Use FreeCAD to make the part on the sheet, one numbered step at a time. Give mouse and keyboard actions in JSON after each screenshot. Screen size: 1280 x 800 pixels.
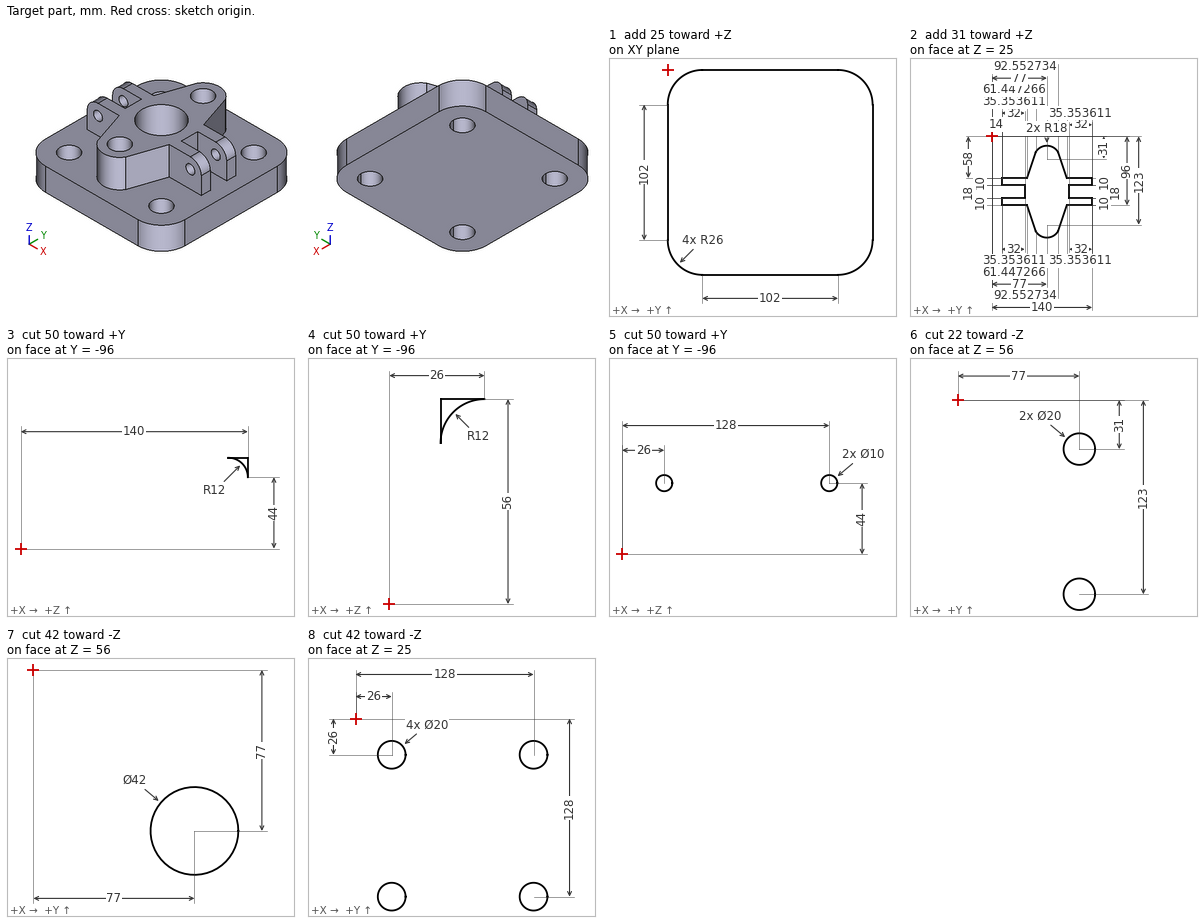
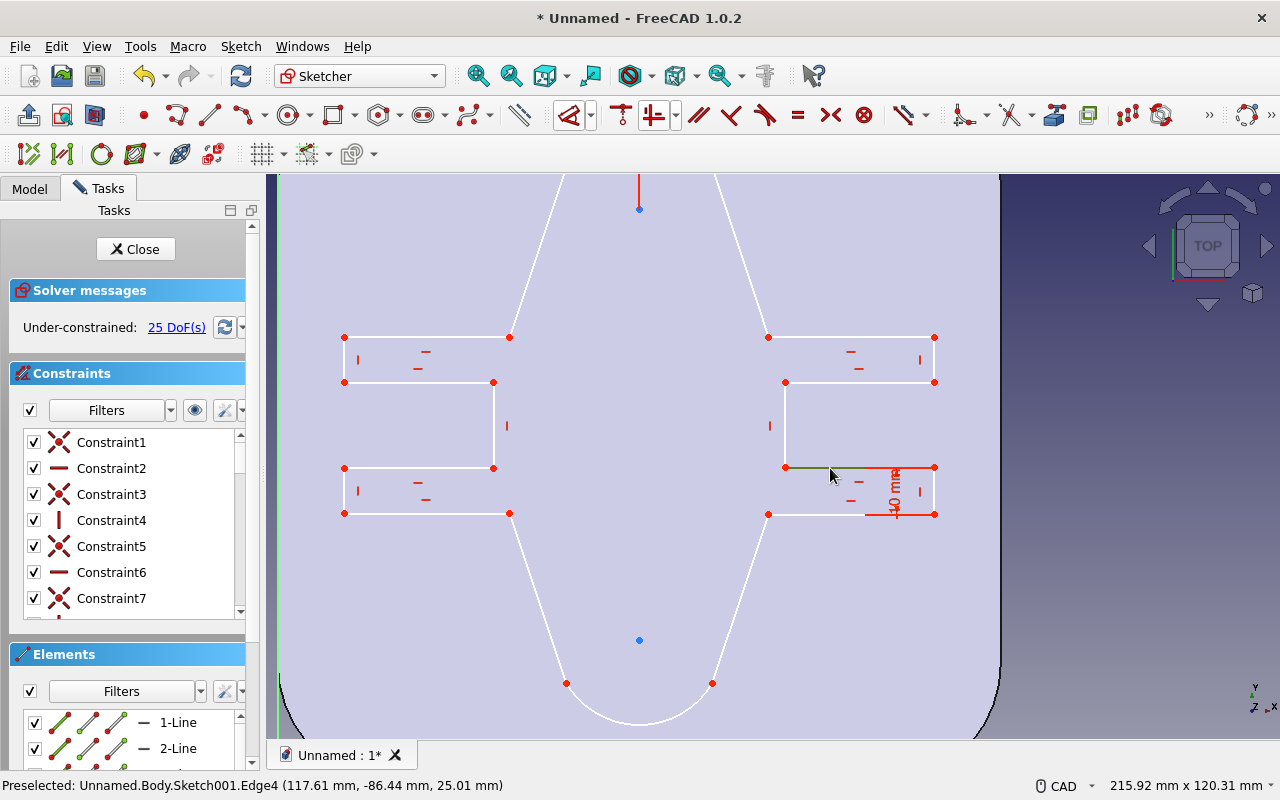
{"action": "key", "text": "l"}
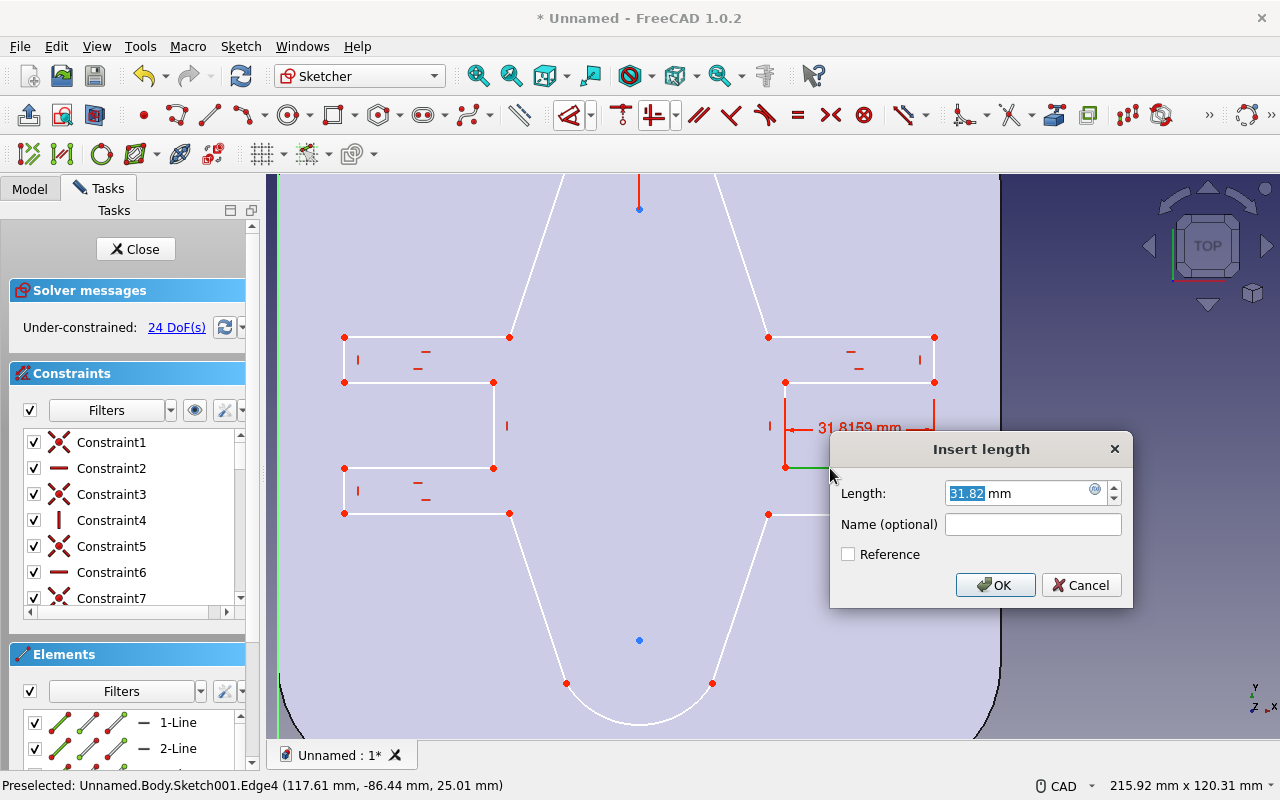
{"action": "type", "text": "32"}
{"action": "key", "text": "Return"}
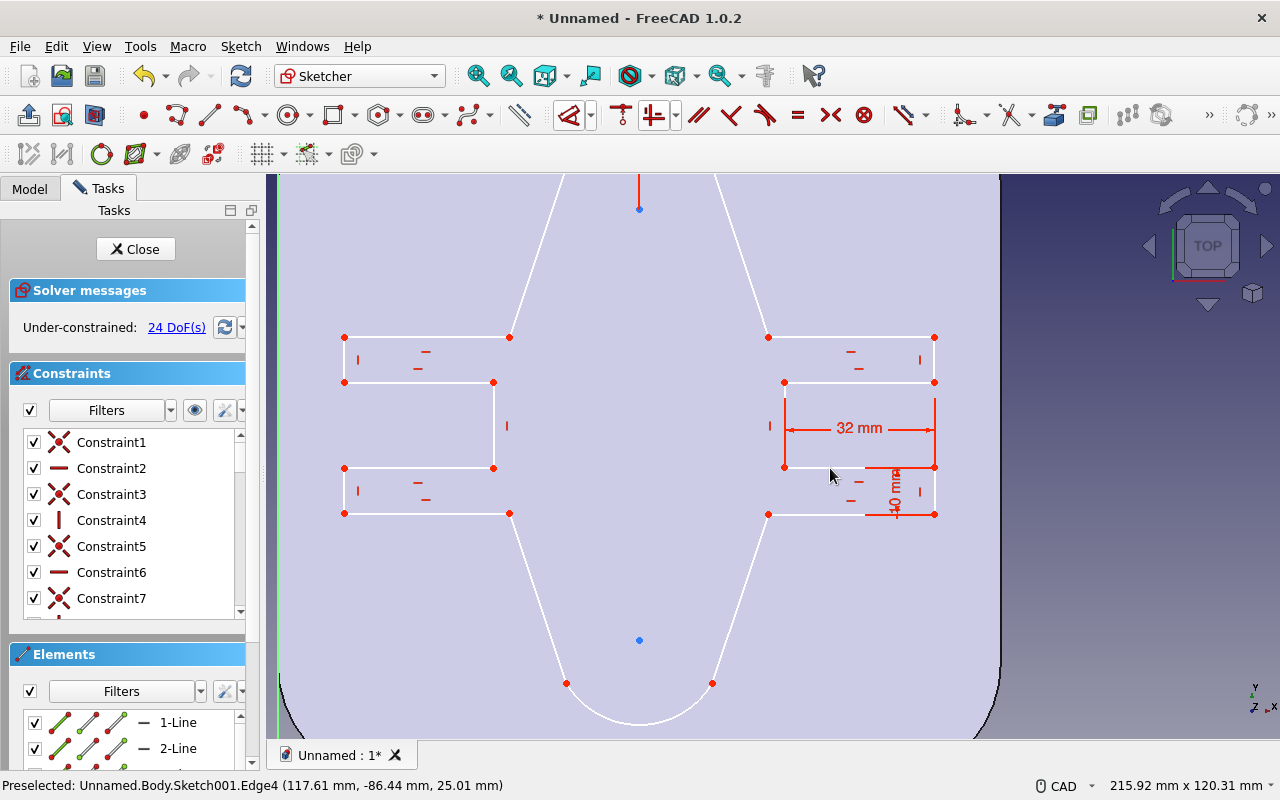
{"action": "left_click", "coordinate": [785, 442]}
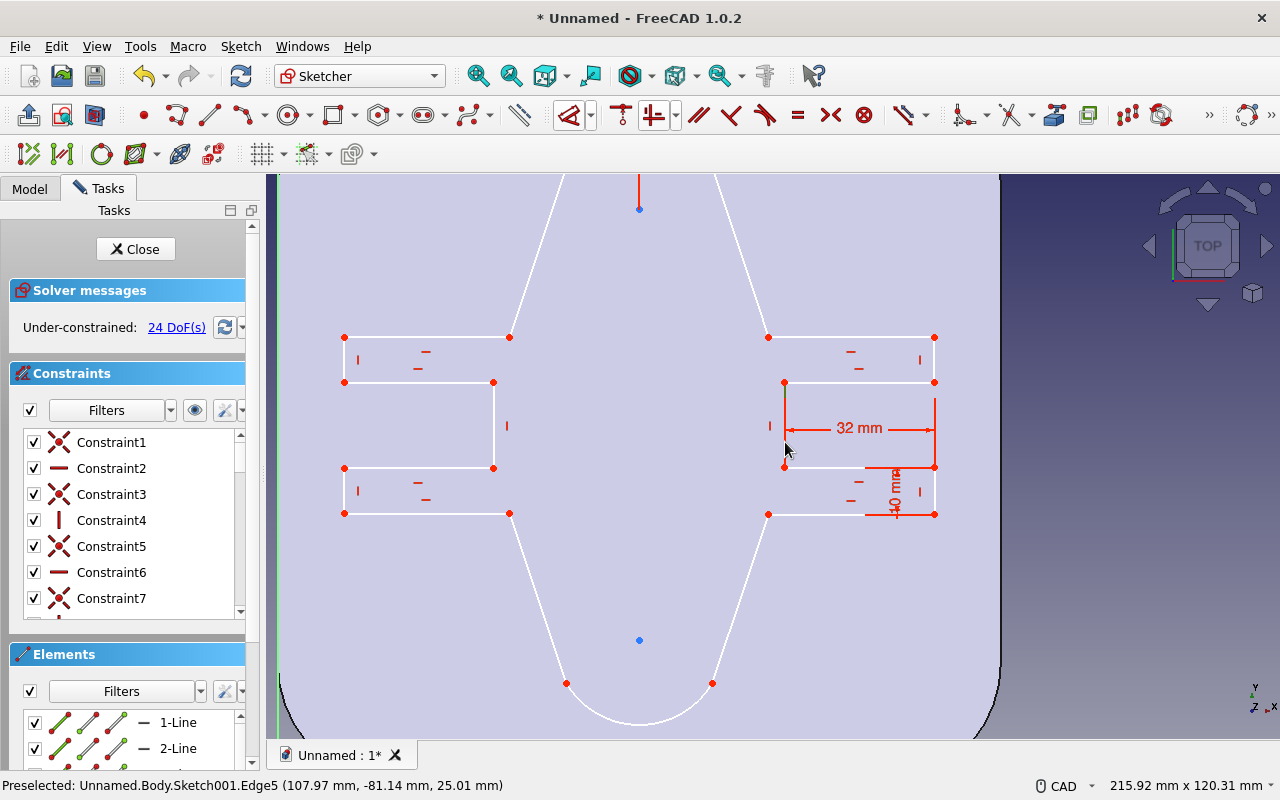
{"action": "left_click", "coordinate": [590, 116]}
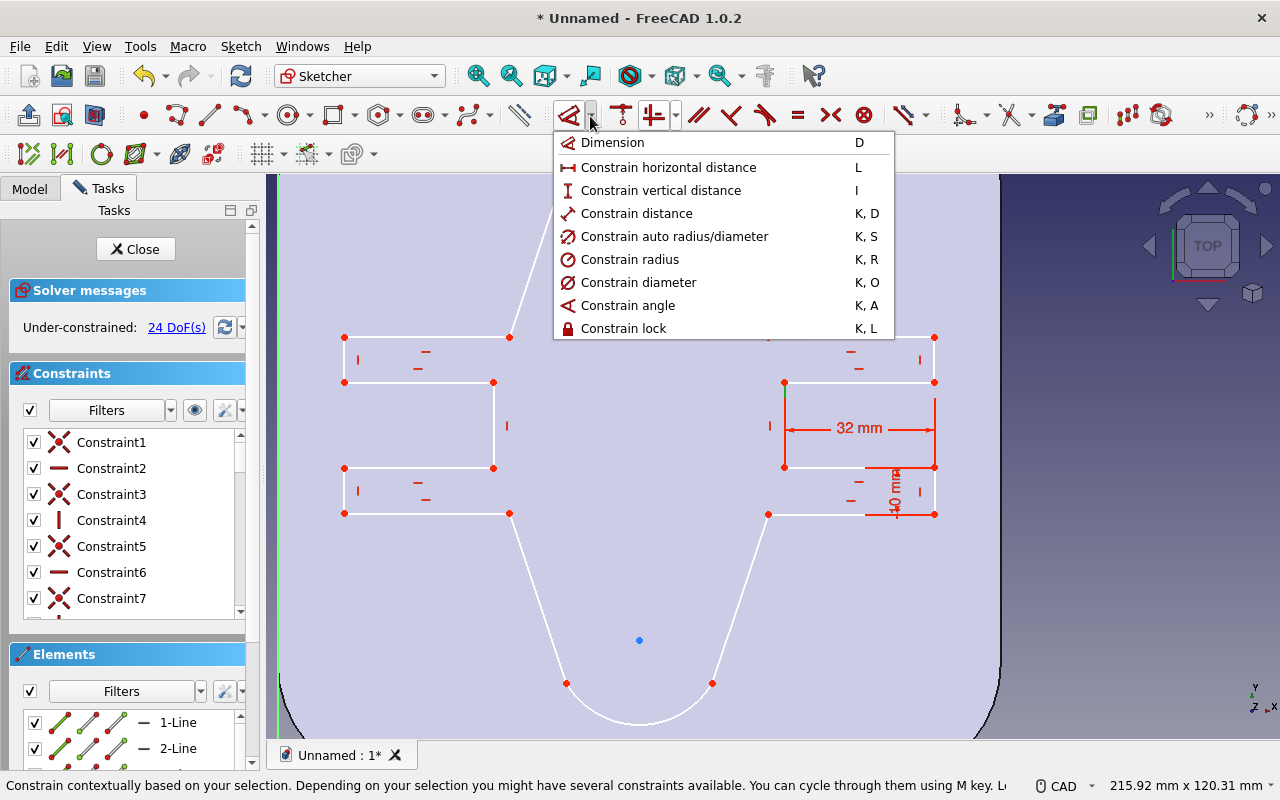
{"action": "left_click", "coordinate": [724, 190]}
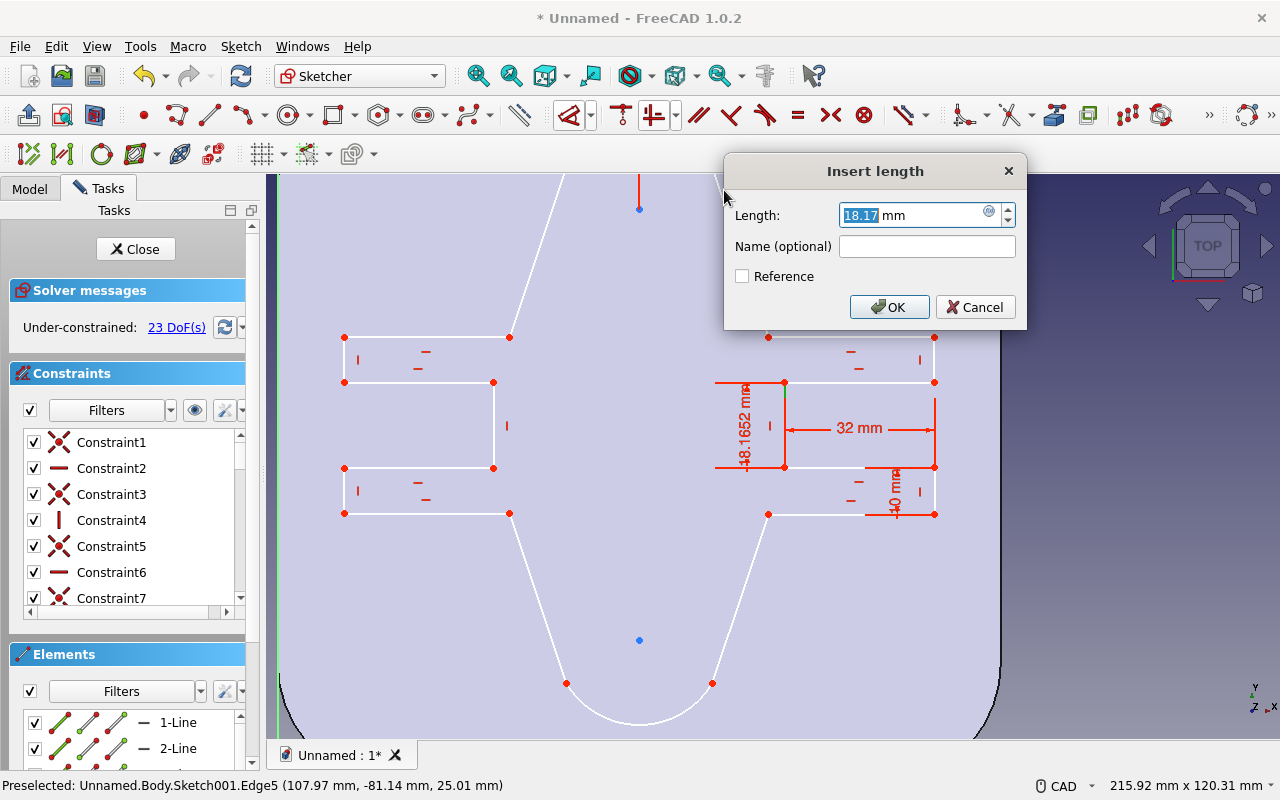
{"action": "type", "text": "18"}
{"action": "key", "text": "Return"}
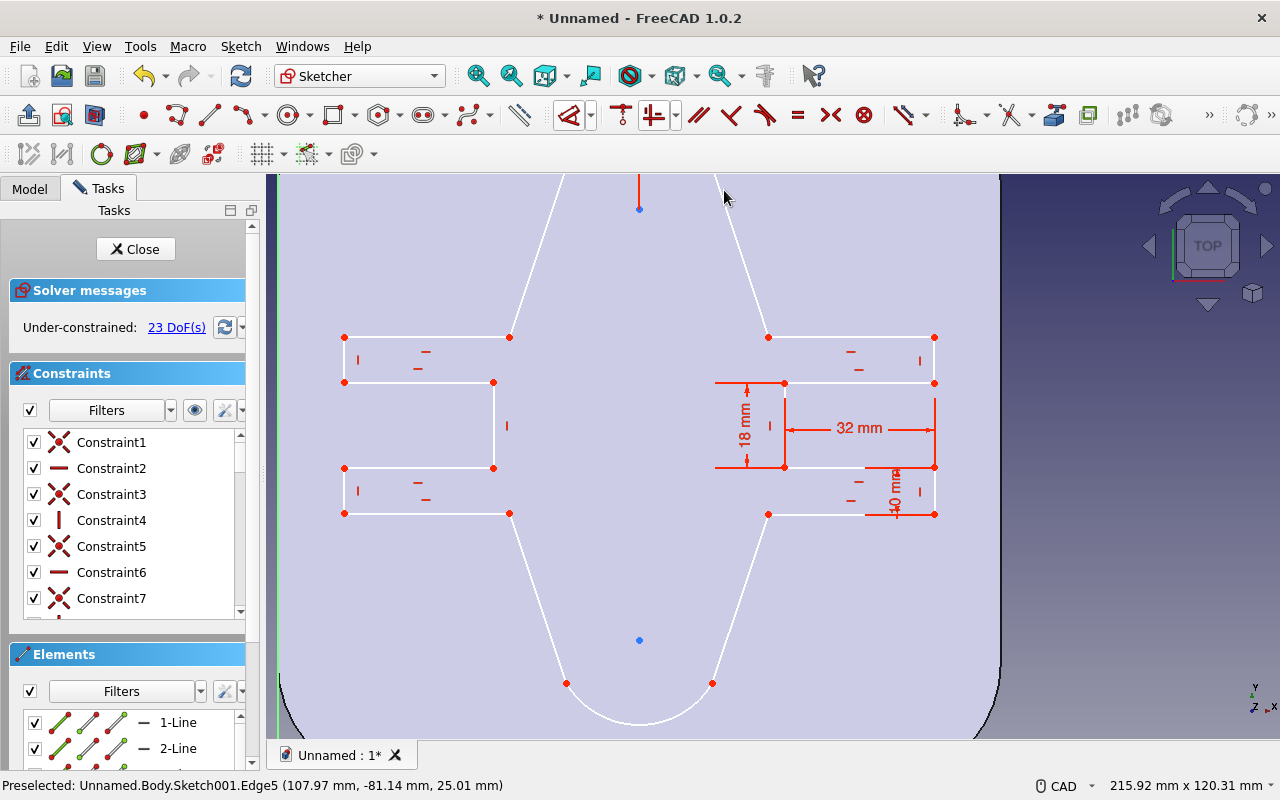
{"action": "left_click", "coordinate": [830, 383]}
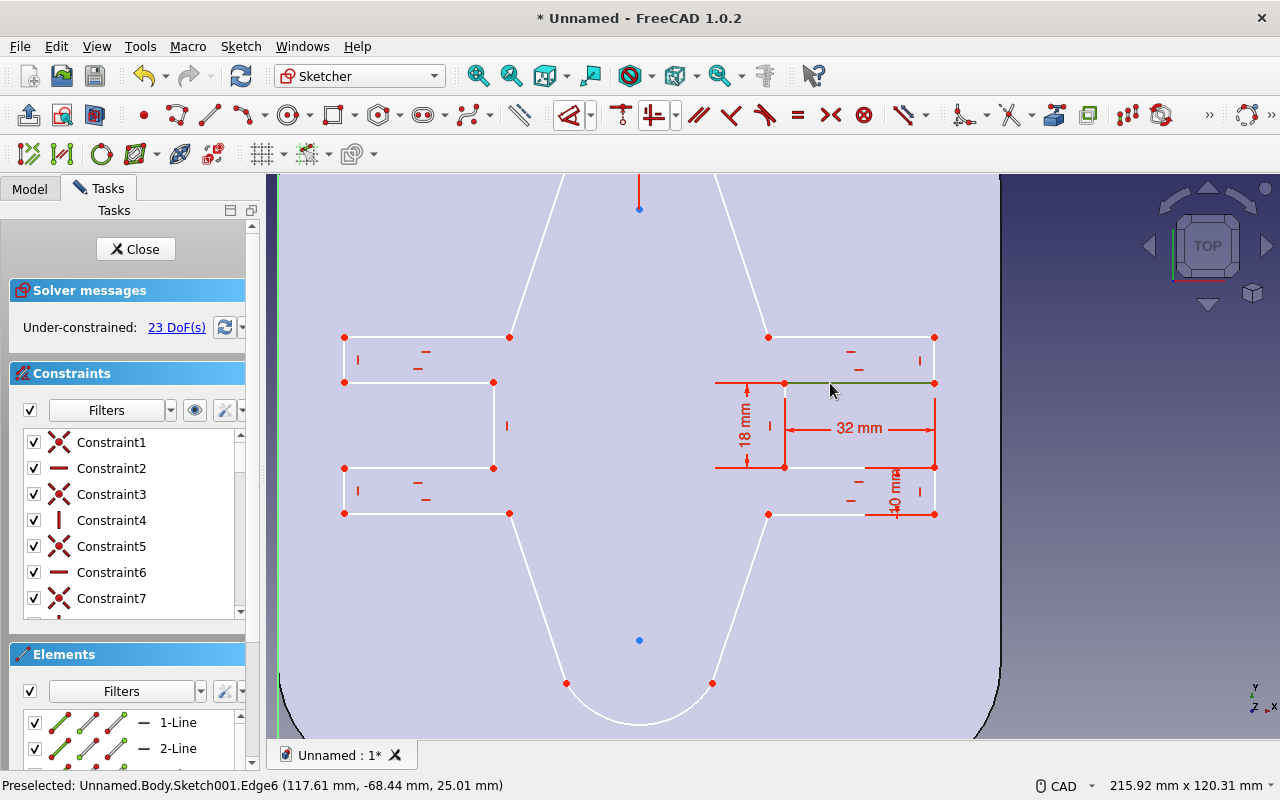
{"action": "key", "text": "l"}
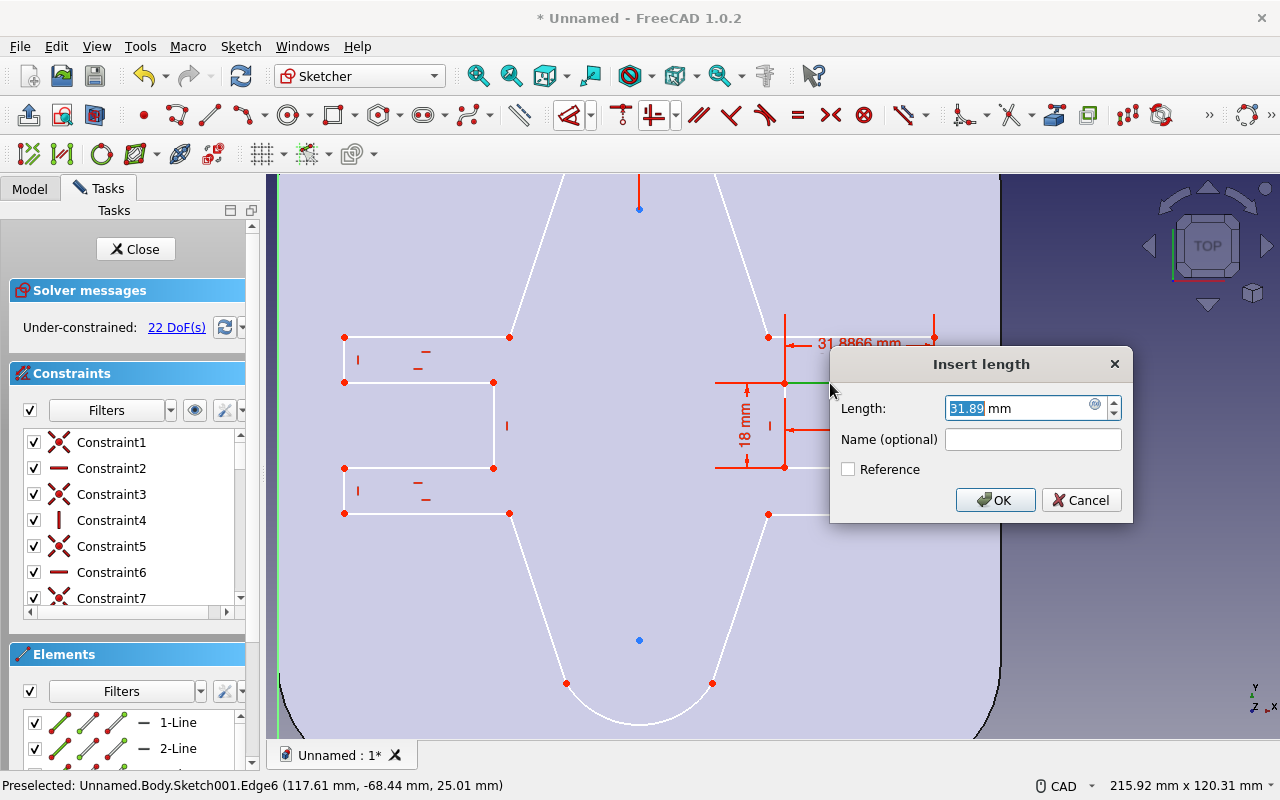
{"action": "type", "text": "32"}
{"action": "key", "text": "Return"}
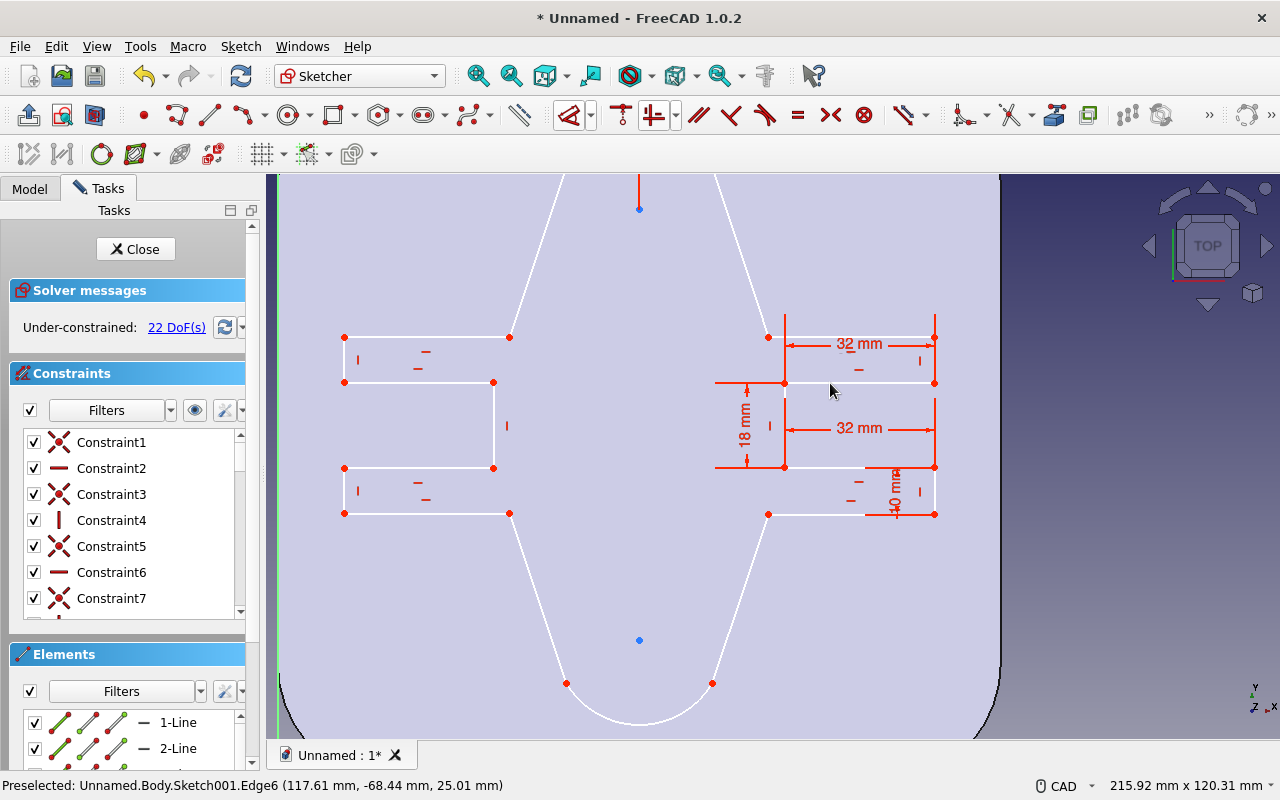
{"action": "left_click", "coordinate": [935, 369]}